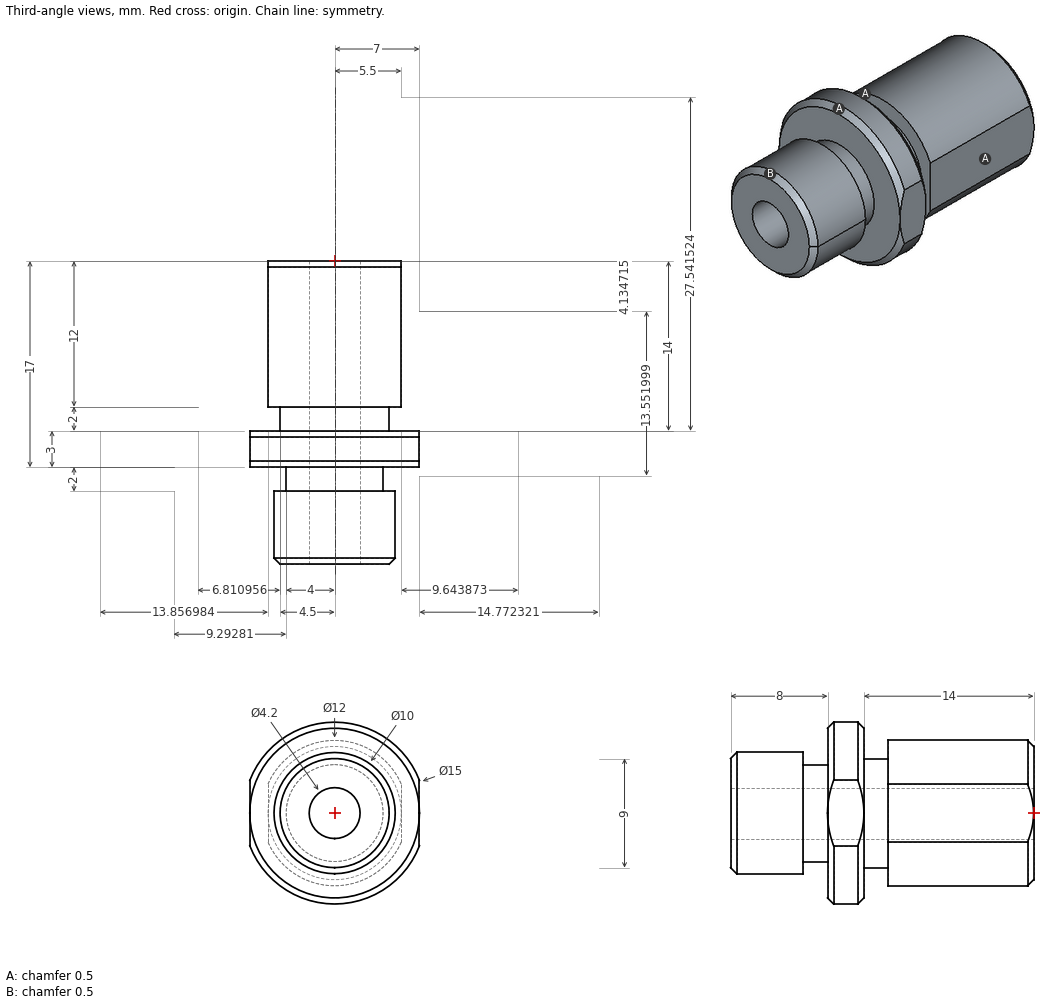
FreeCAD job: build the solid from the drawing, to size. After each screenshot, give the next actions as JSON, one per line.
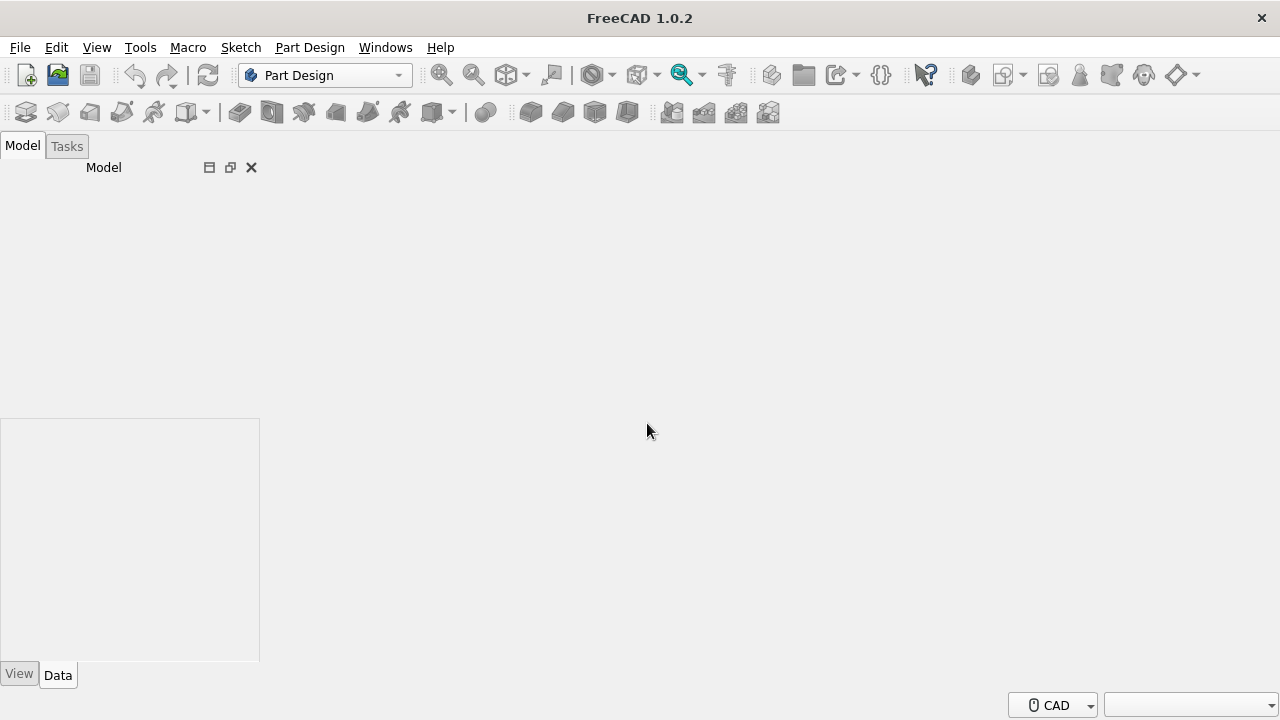
{"action": "left_click", "coordinate": [26, 76]}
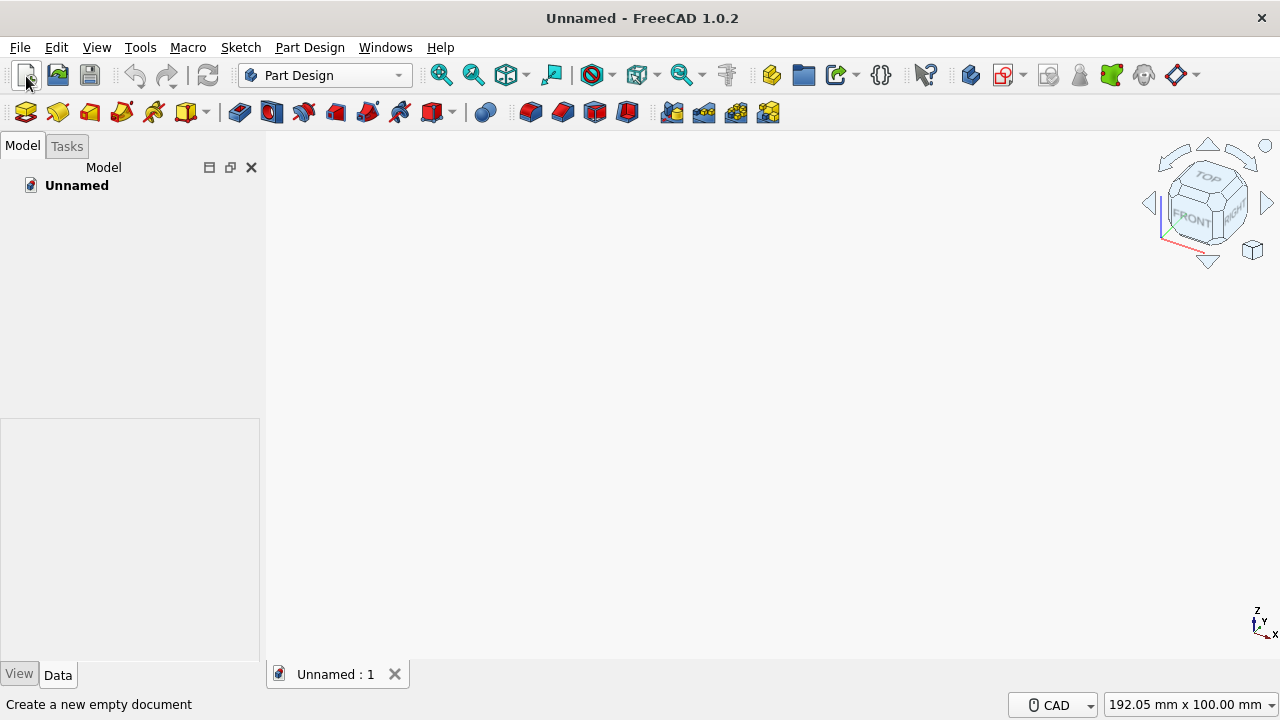
{"action": "left_click", "coordinate": [1004, 76]}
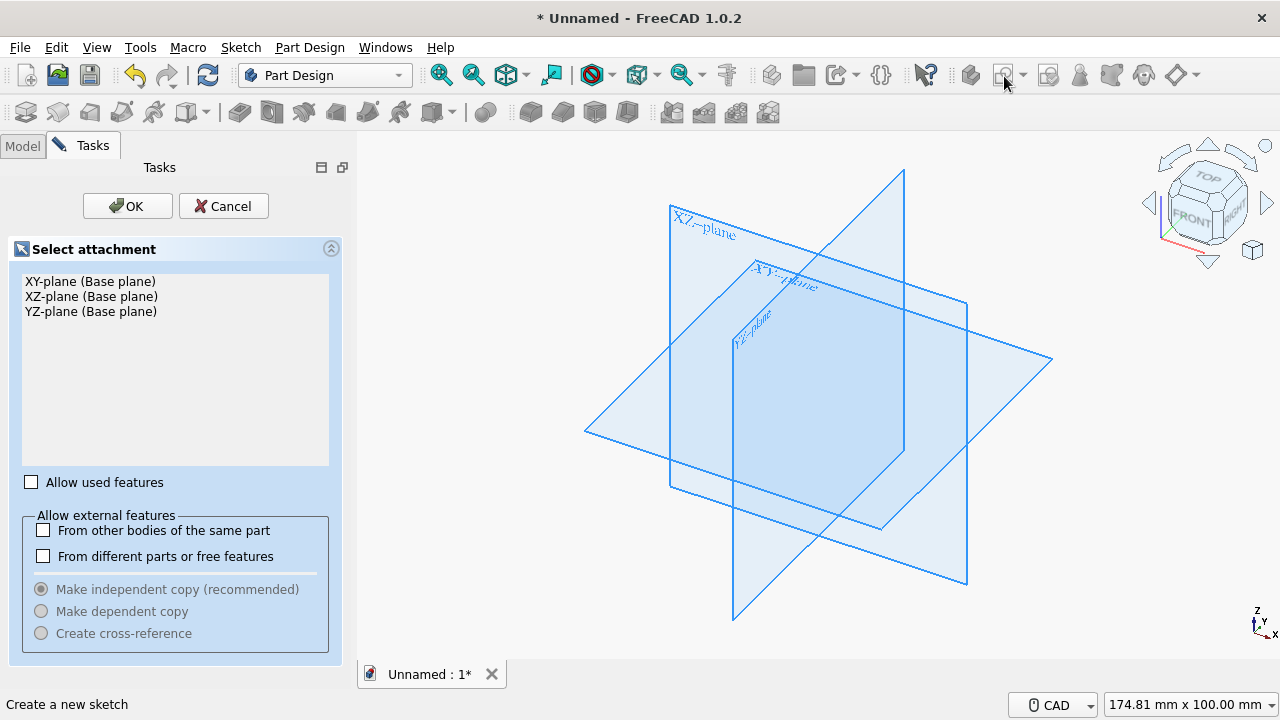
{"action": "left_click", "coordinate": [82, 296]}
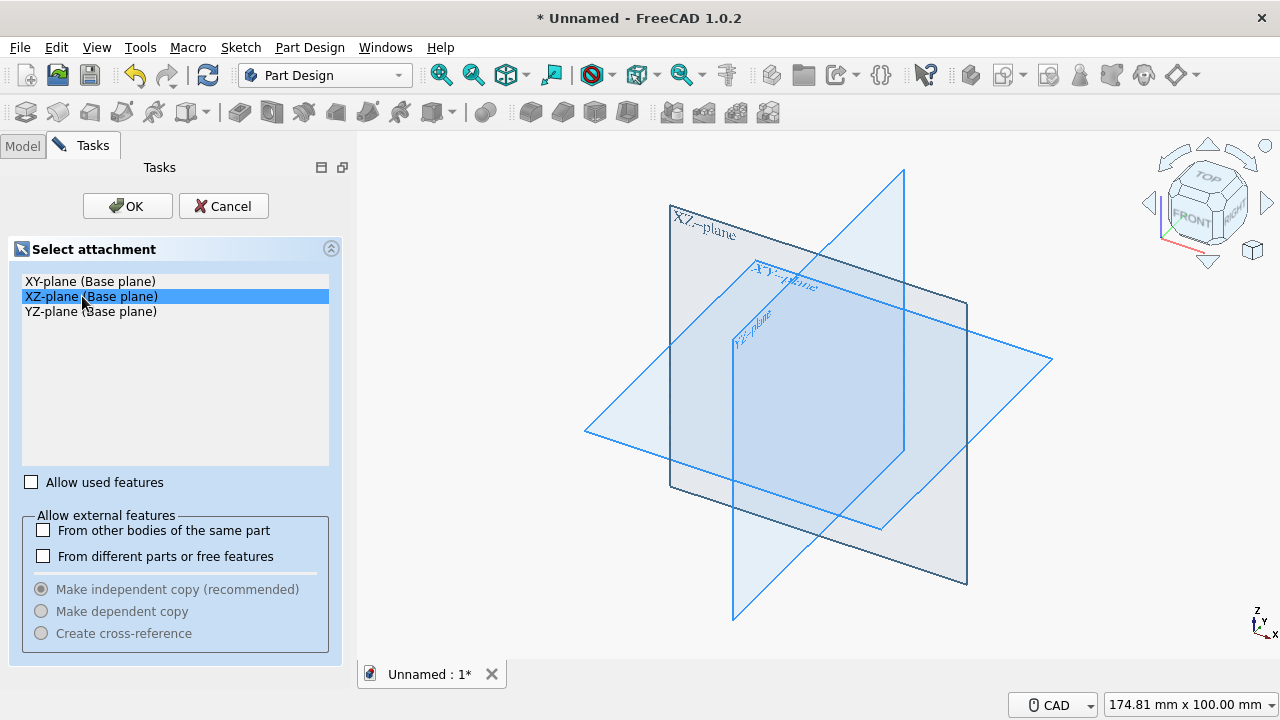
{"action": "left_click", "coordinate": [128, 206]}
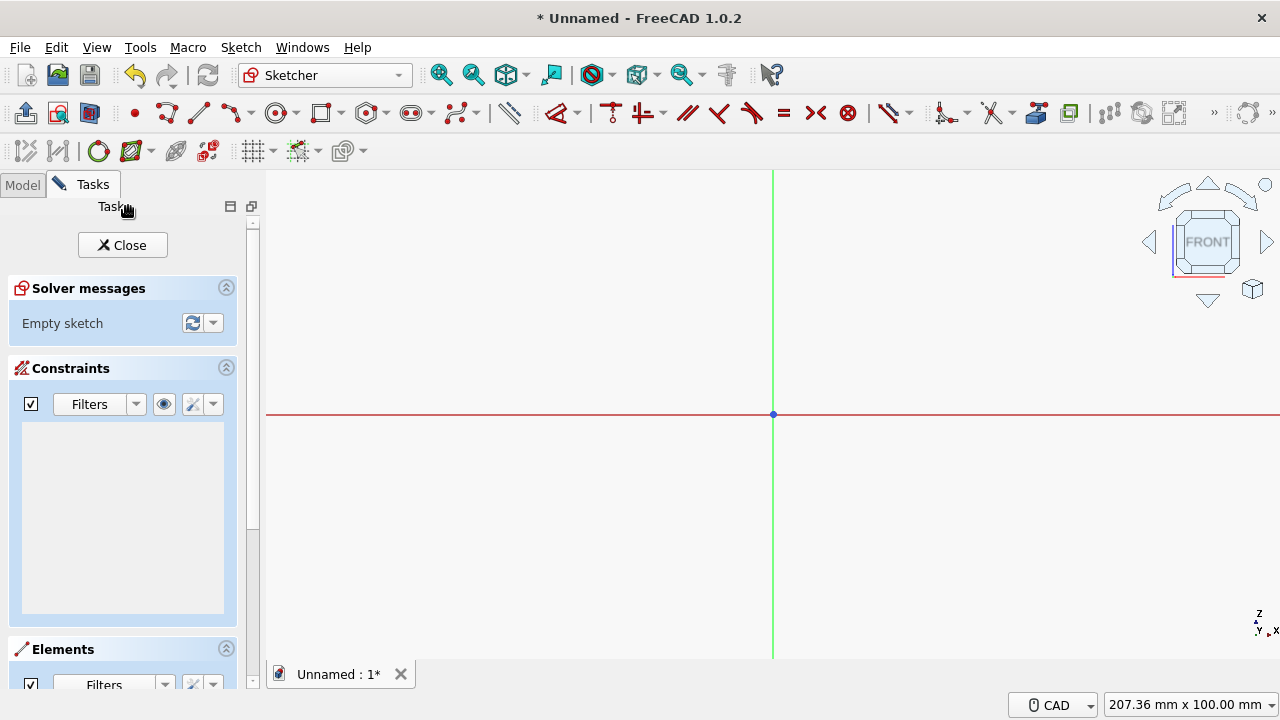
{"action": "scroll", "coordinate": [790, 414], "scroll_direction": "up", "scroll_amount": 8}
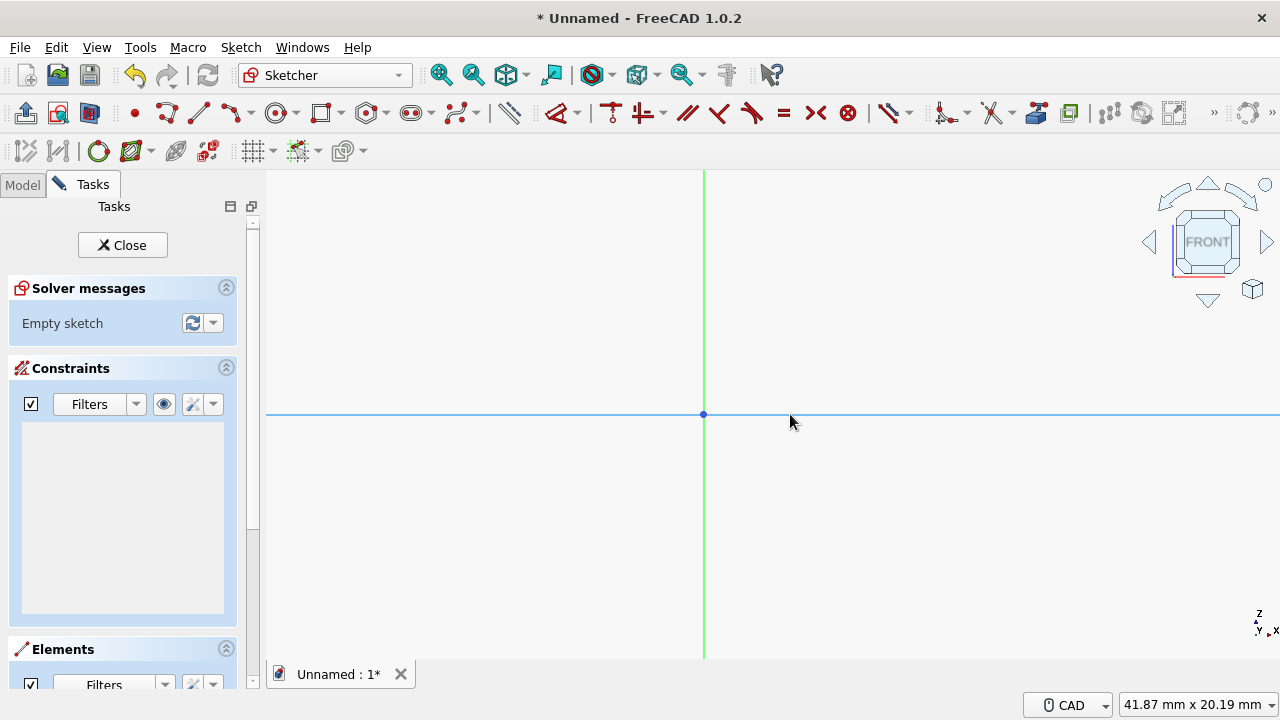
{"action": "key", "text": "g c"}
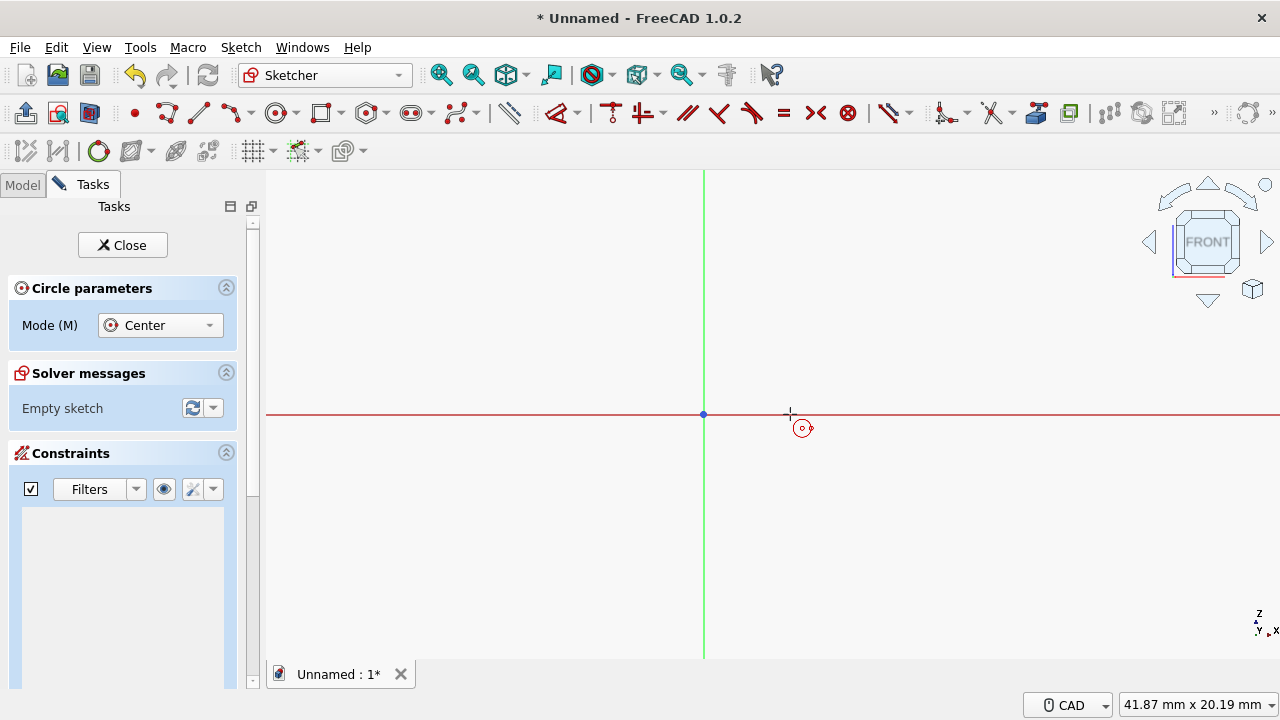
{"action": "left_click", "coordinate": [704, 414]}
{"action": "left_click", "coordinate": [807, 312]}
{"action": "key", "text": "Escape"}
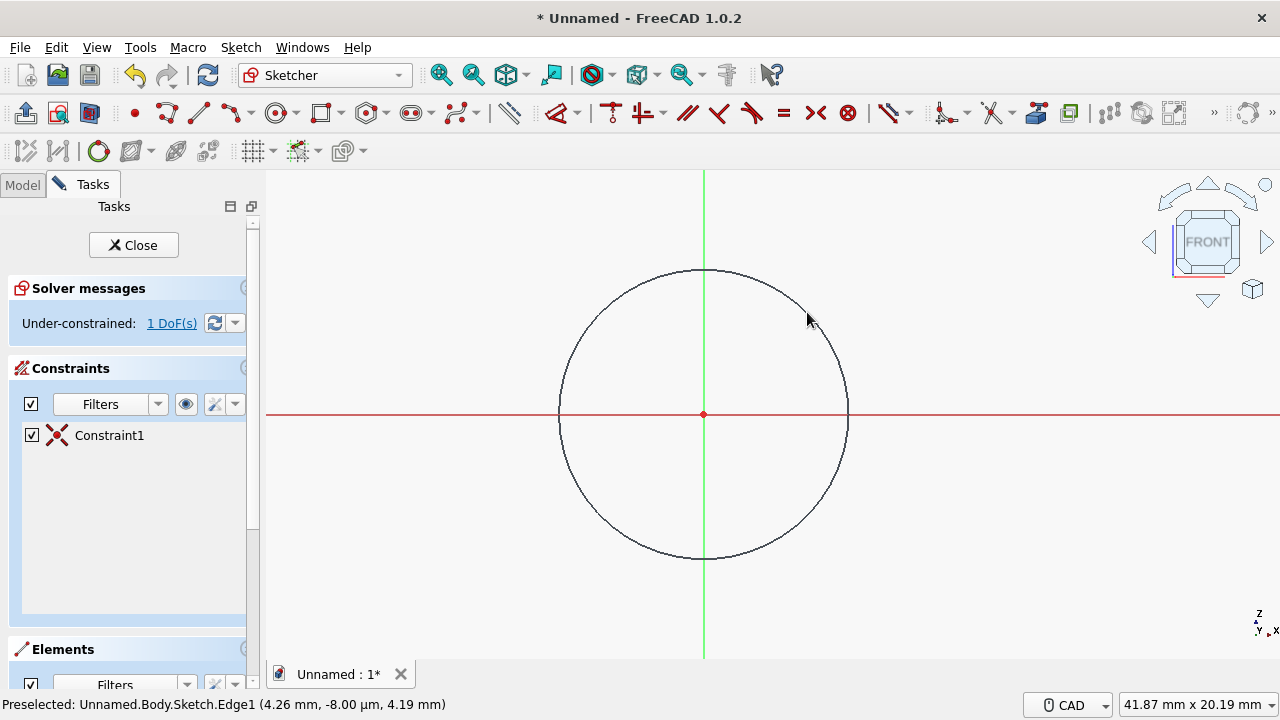
{"action": "left_click", "coordinate": [556, 114]}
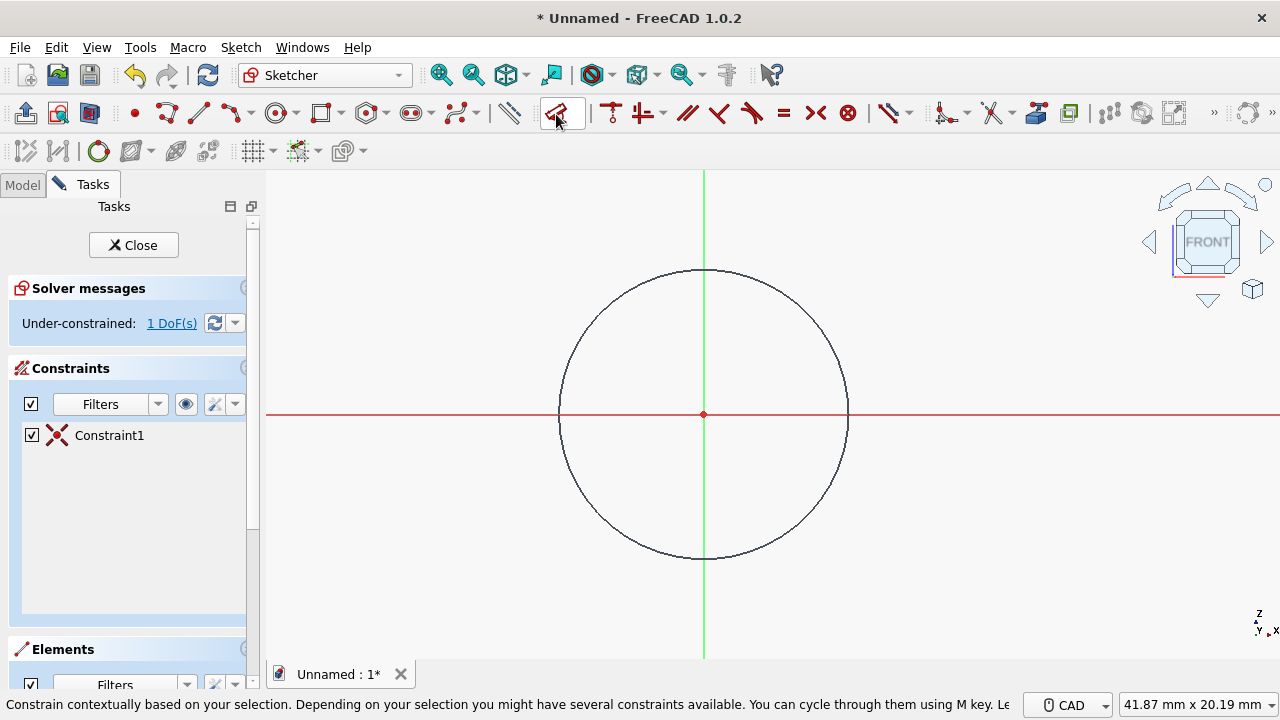
{"action": "left_click", "coordinate": [806, 312]}
{"action": "left_click", "coordinate": [829, 289]}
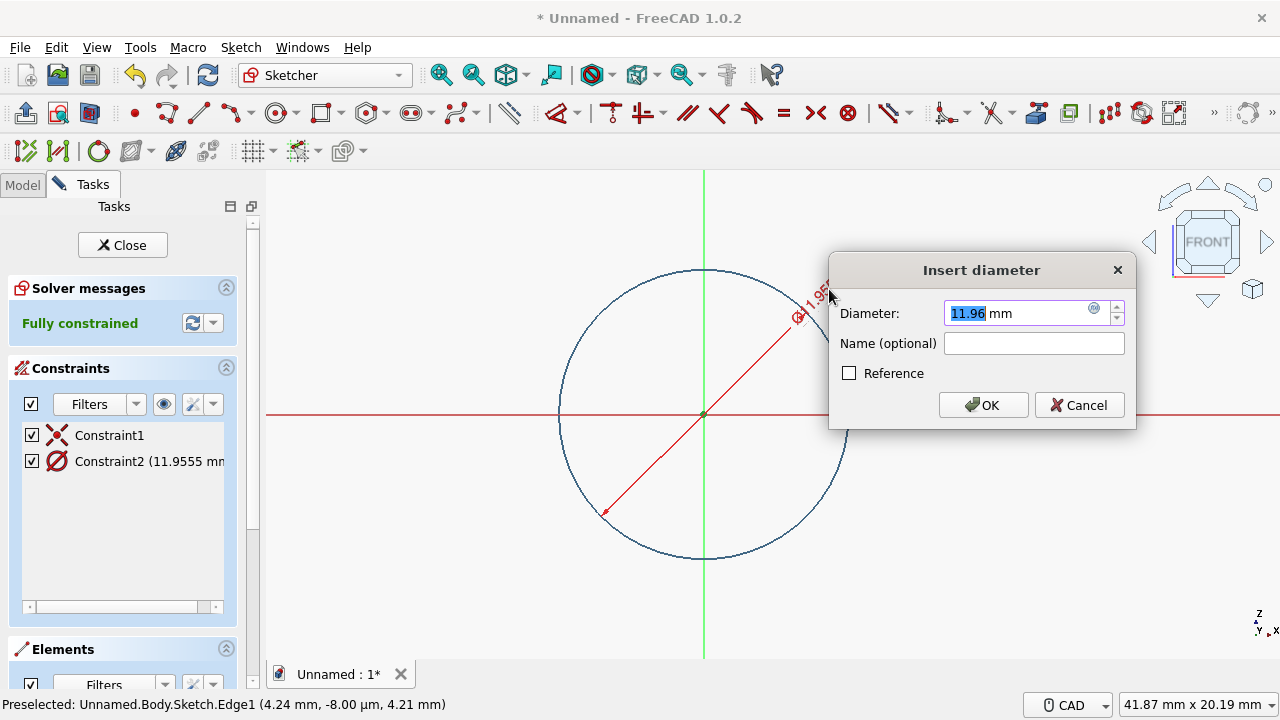
{"action": "type", "text": "12"}
{"action": "key", "text": "Return"}
{"action": "key", "text": "Escape"}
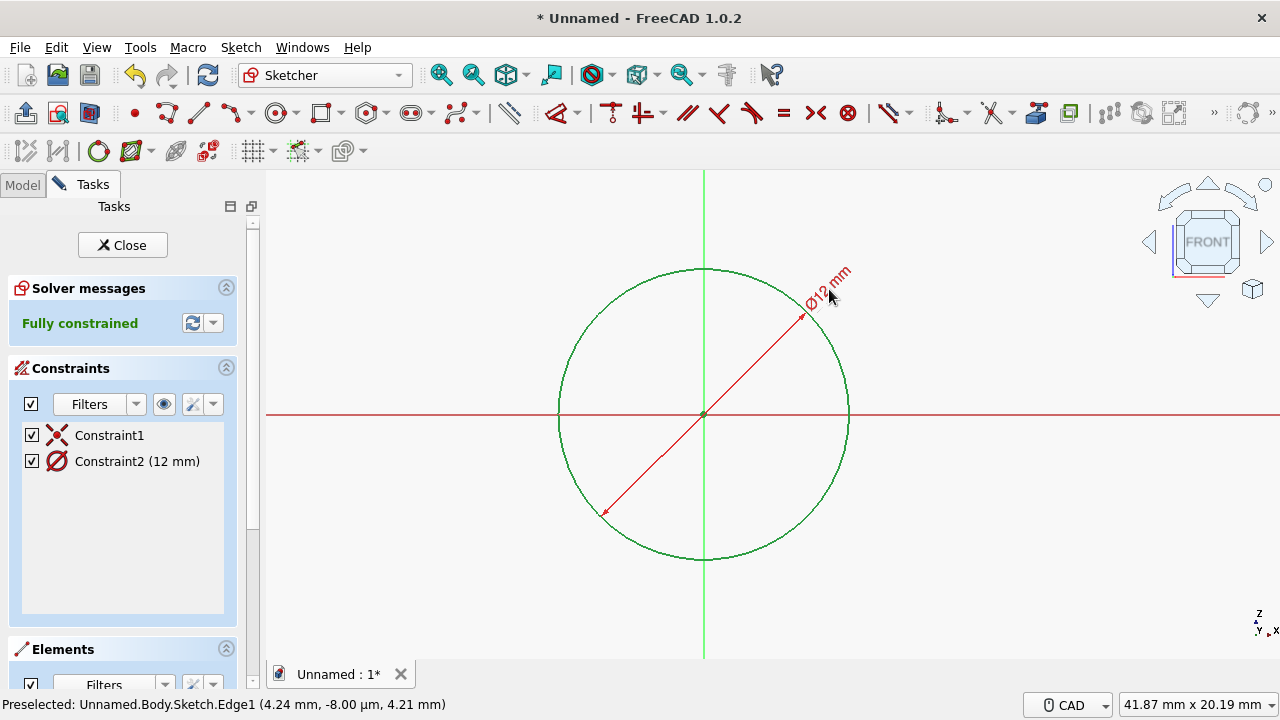
{"action": "left_click", "coordinate": [123, 245]}